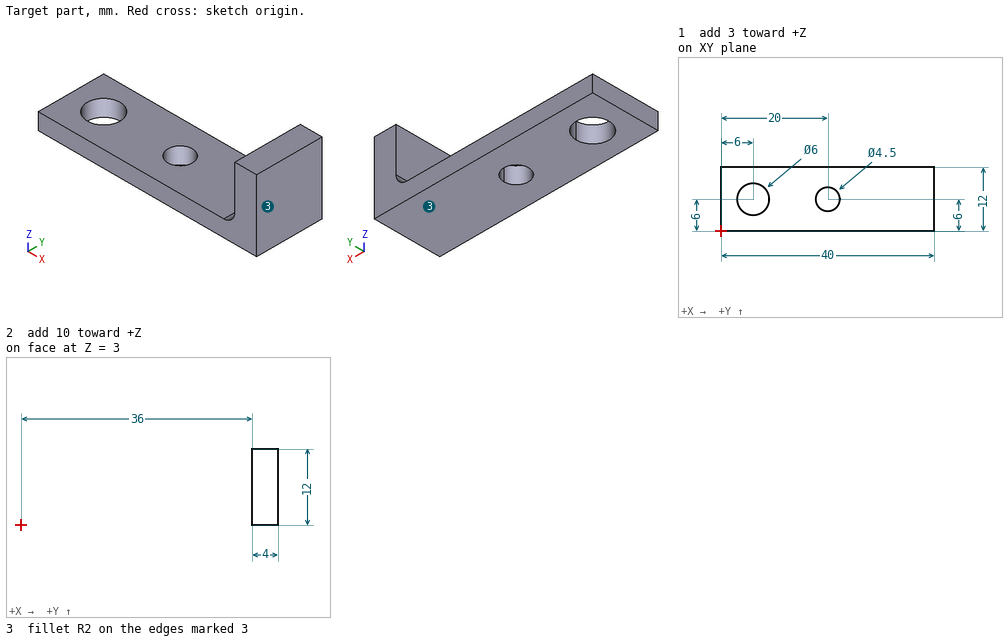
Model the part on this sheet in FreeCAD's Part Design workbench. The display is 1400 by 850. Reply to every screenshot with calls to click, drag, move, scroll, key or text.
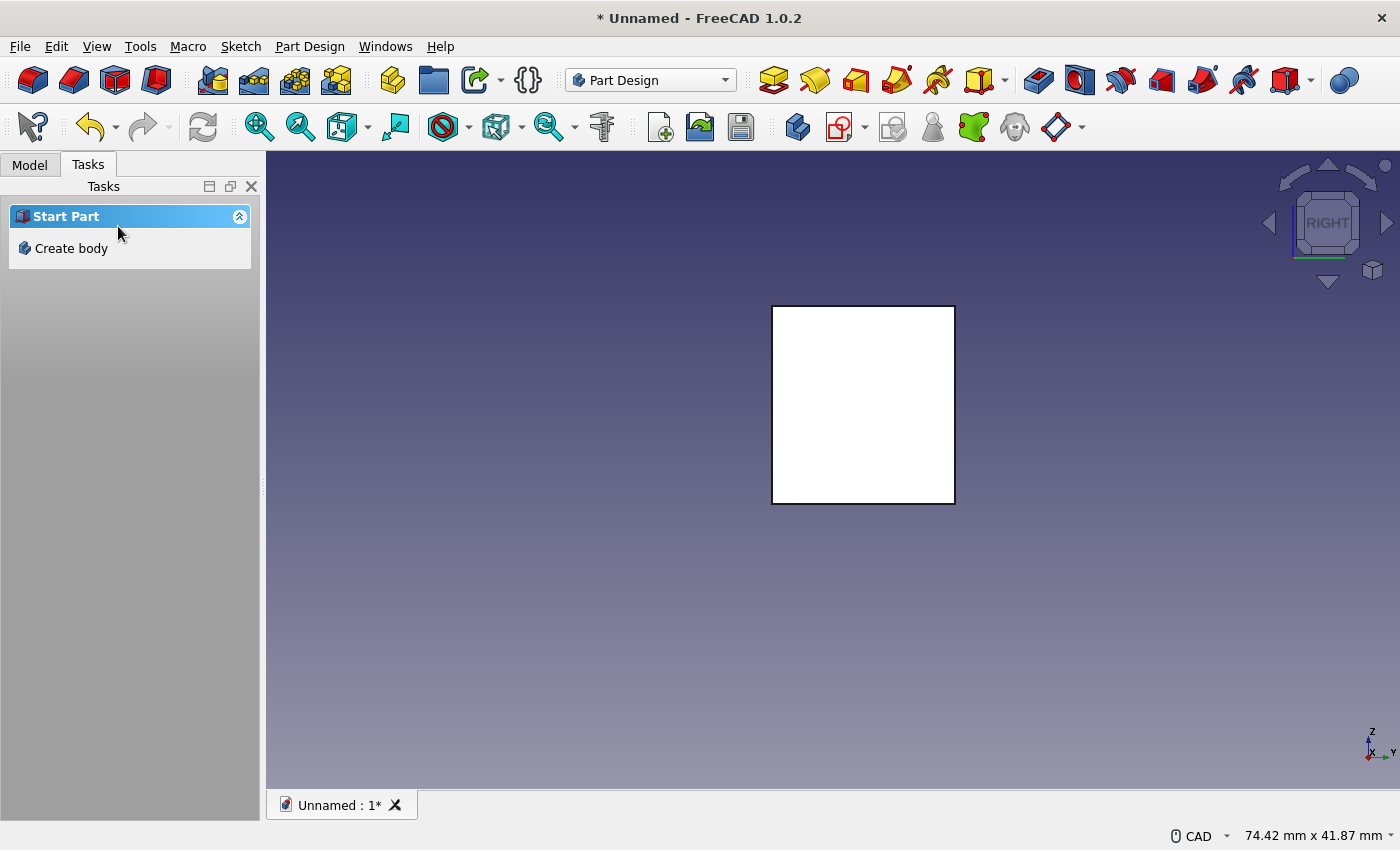
click(260, 128)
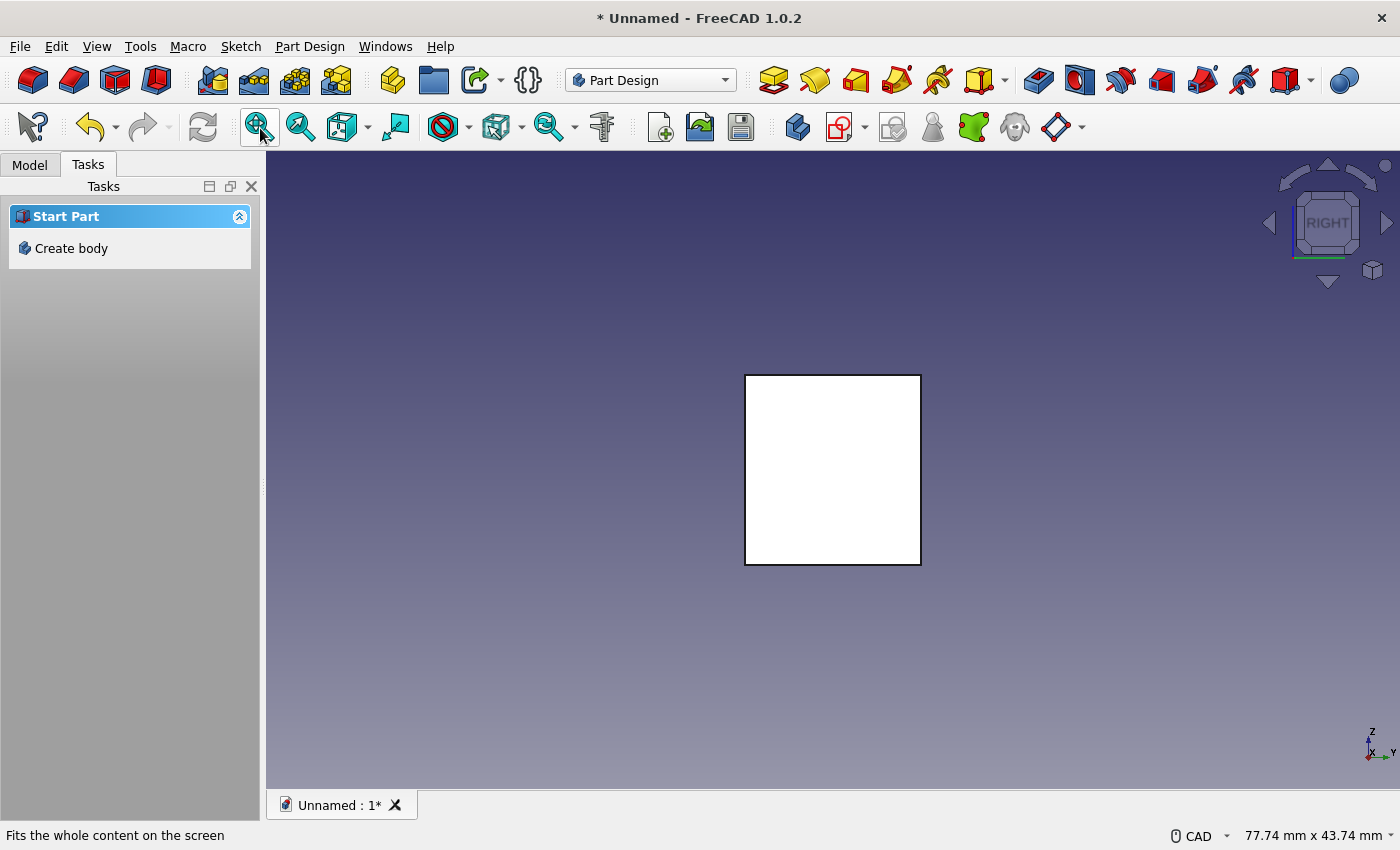
key(5)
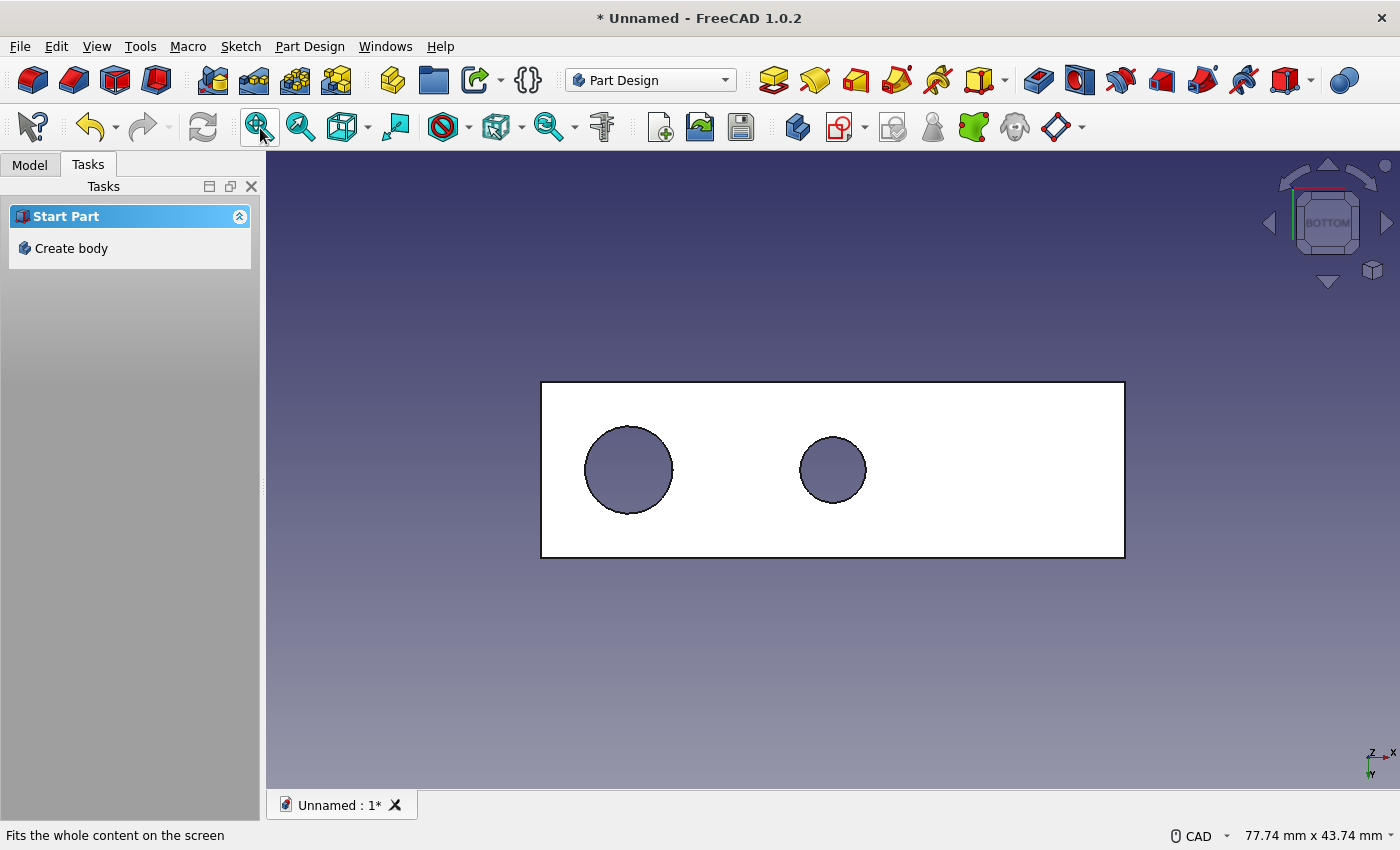
key(4)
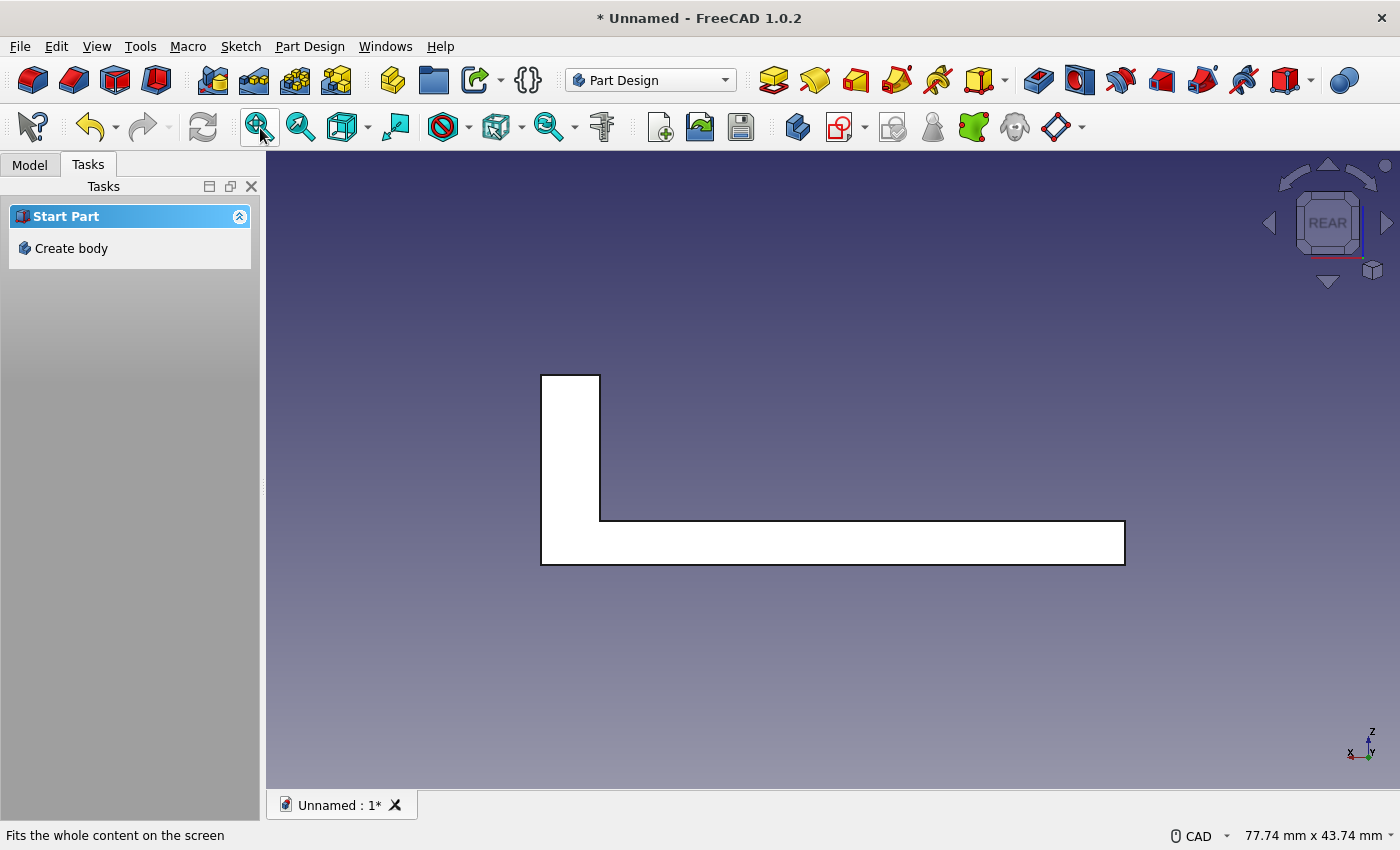
key(6)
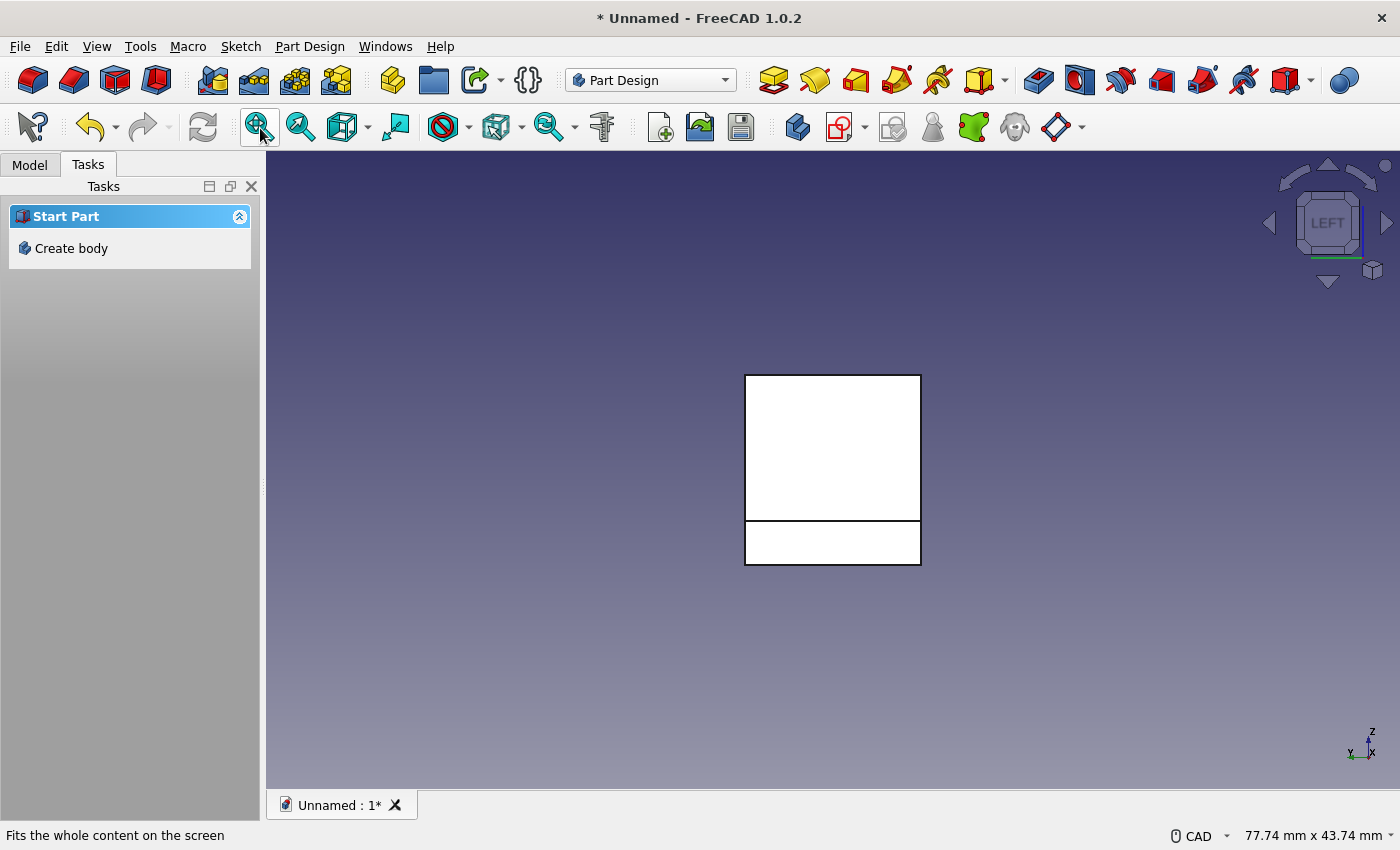
click(260, 128)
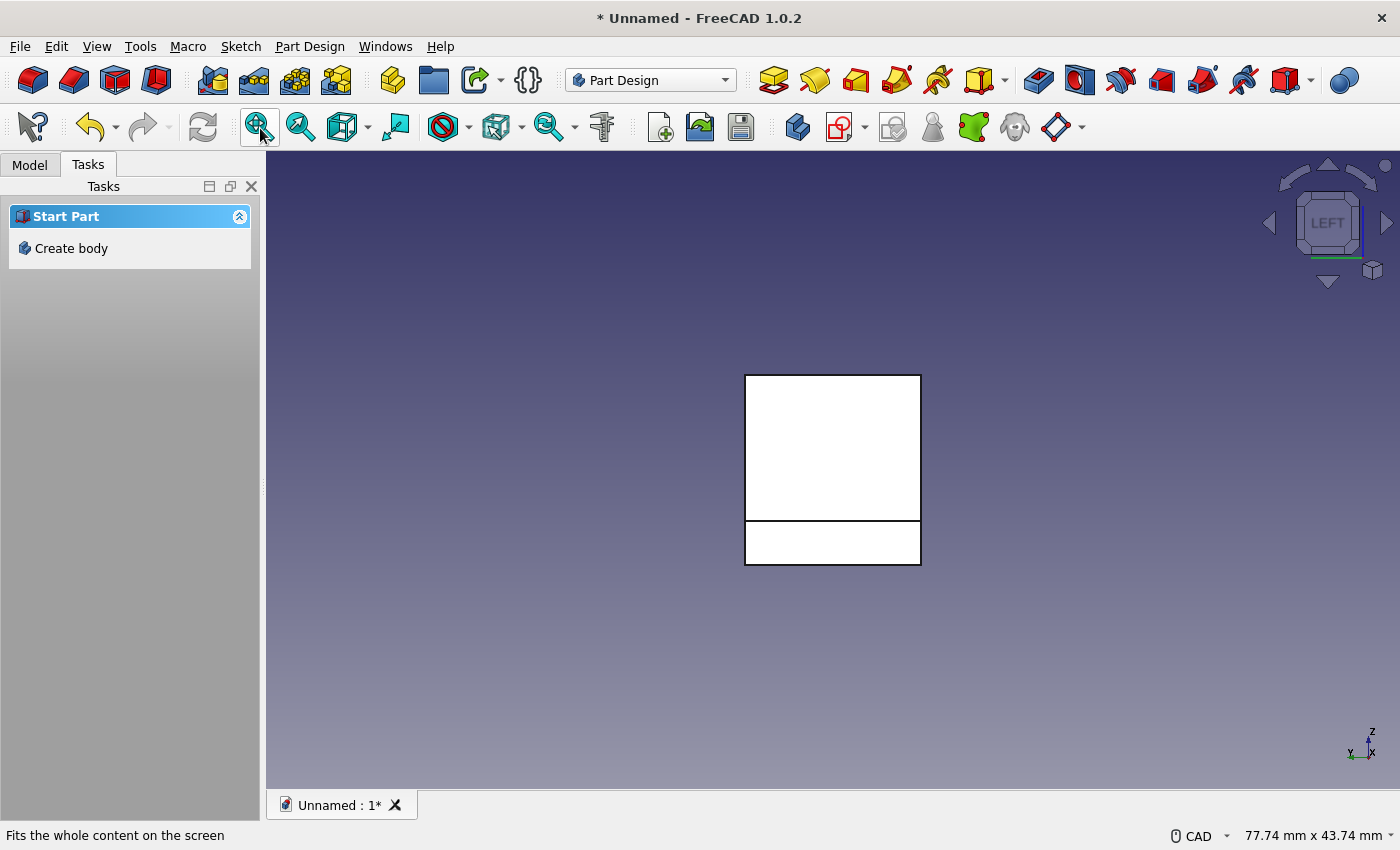
key(v)
key(3)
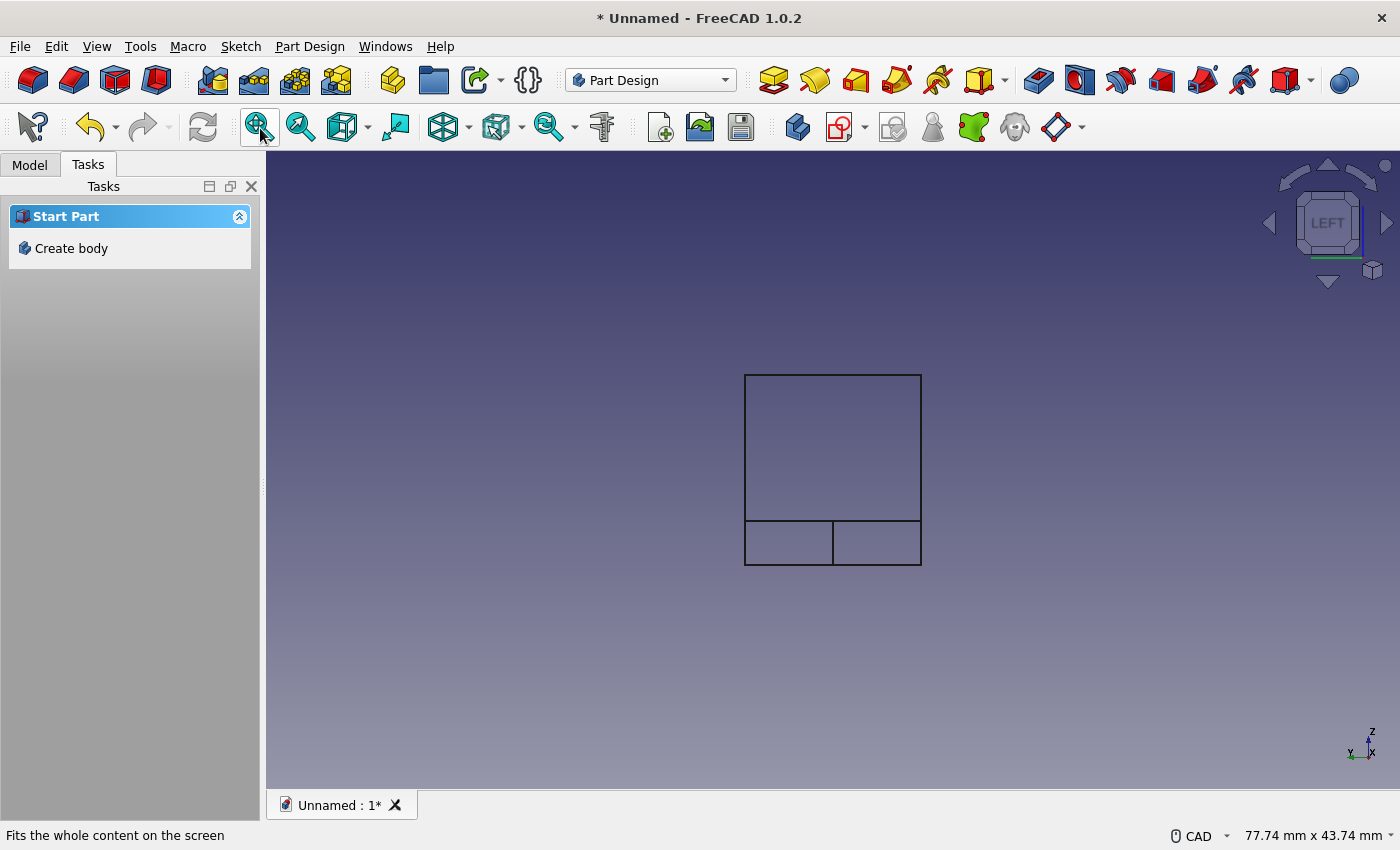
key(0)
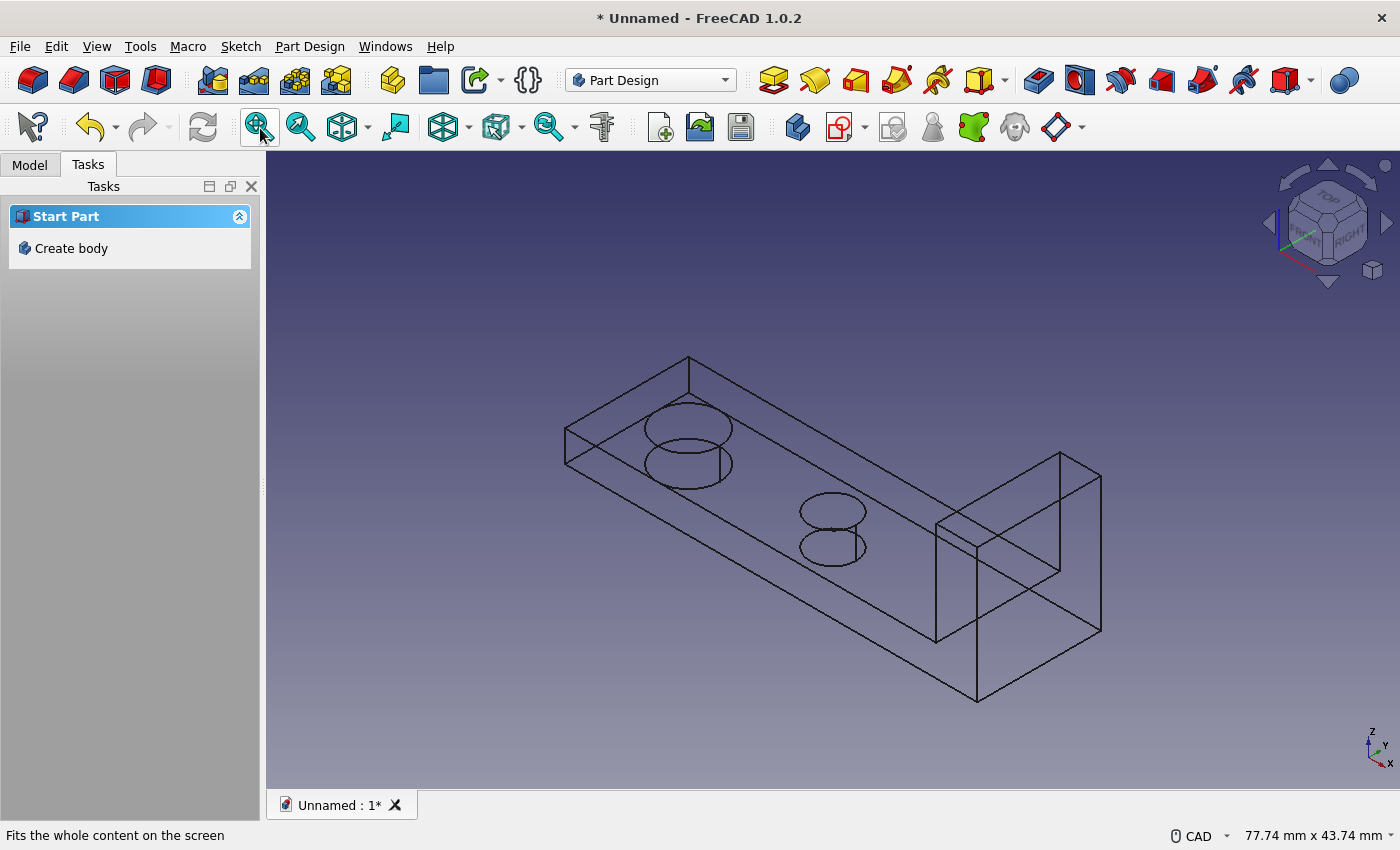
click(998, 606)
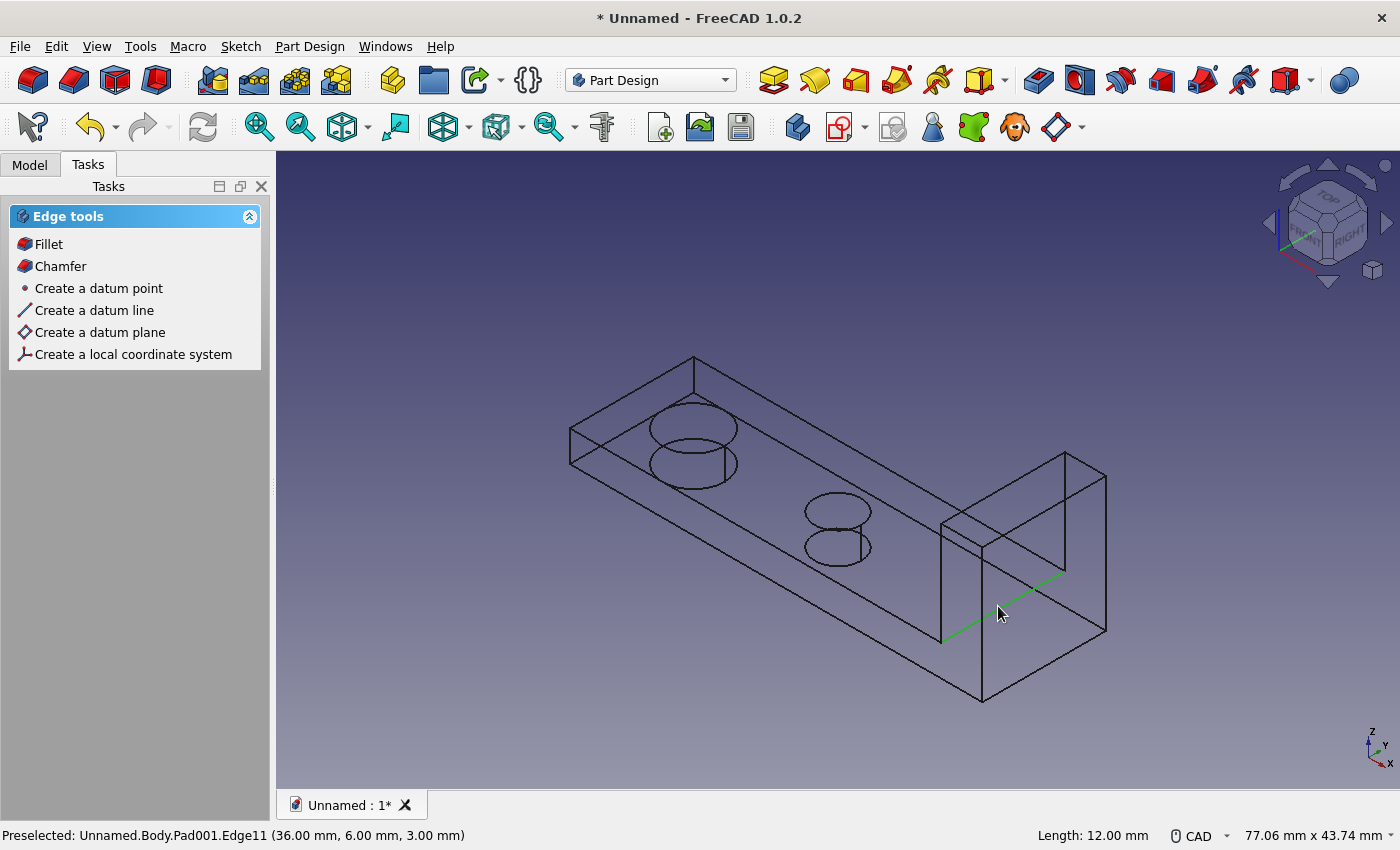
key(v)
key(1)